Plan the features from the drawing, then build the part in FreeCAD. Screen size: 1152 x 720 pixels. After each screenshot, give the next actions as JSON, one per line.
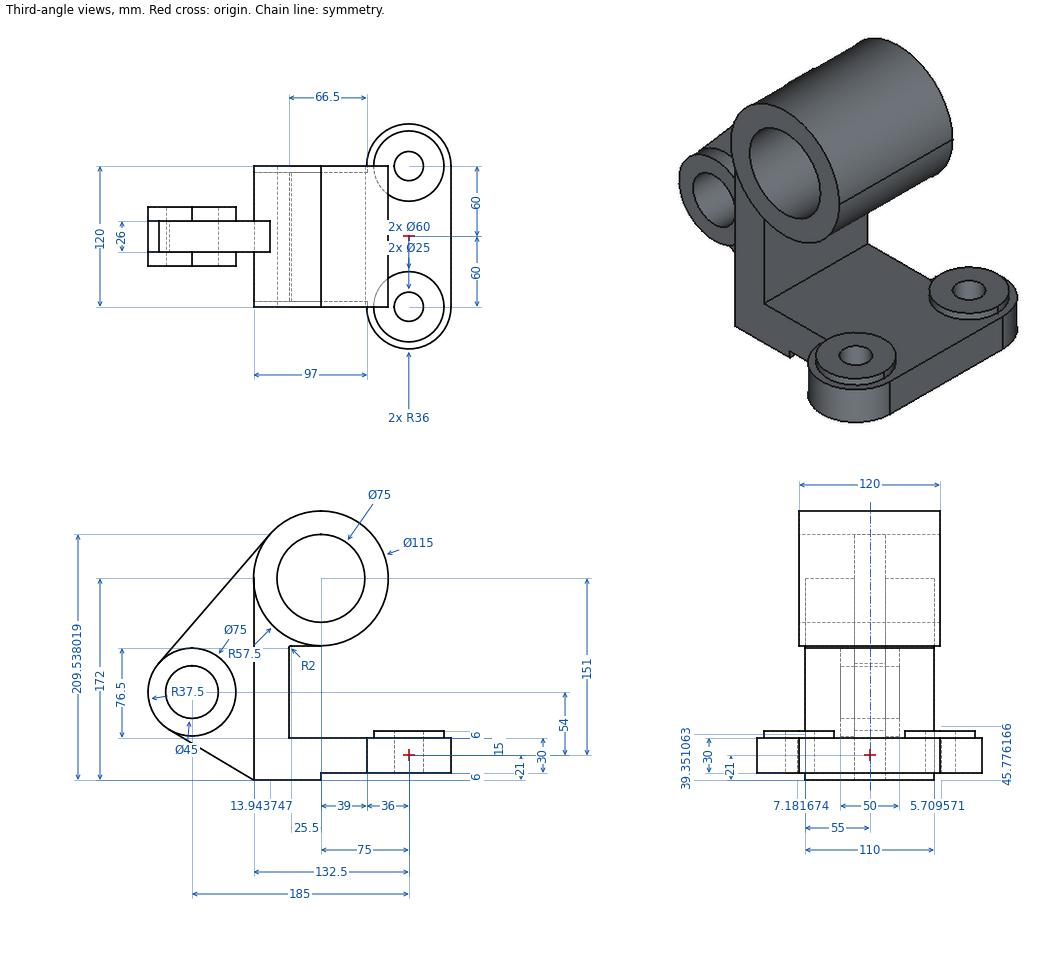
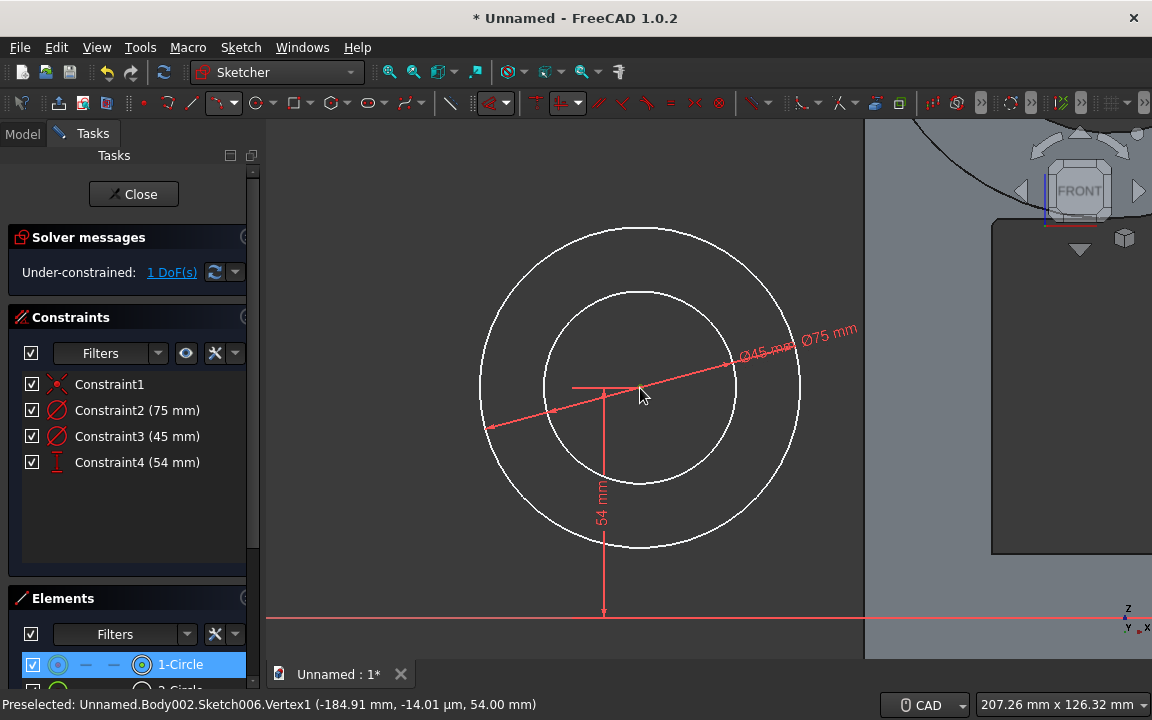
{"action": "key", "text": "l"}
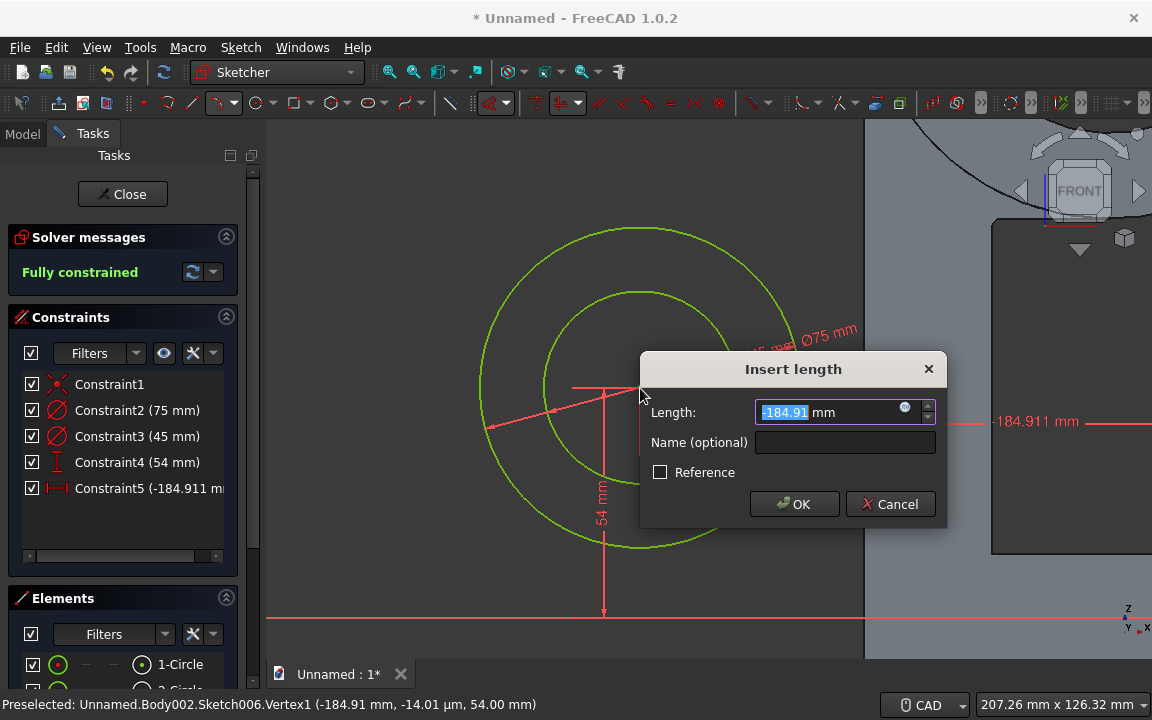
{"action": "type", "text": "-185"}
{"action": "key", "text": "Return"}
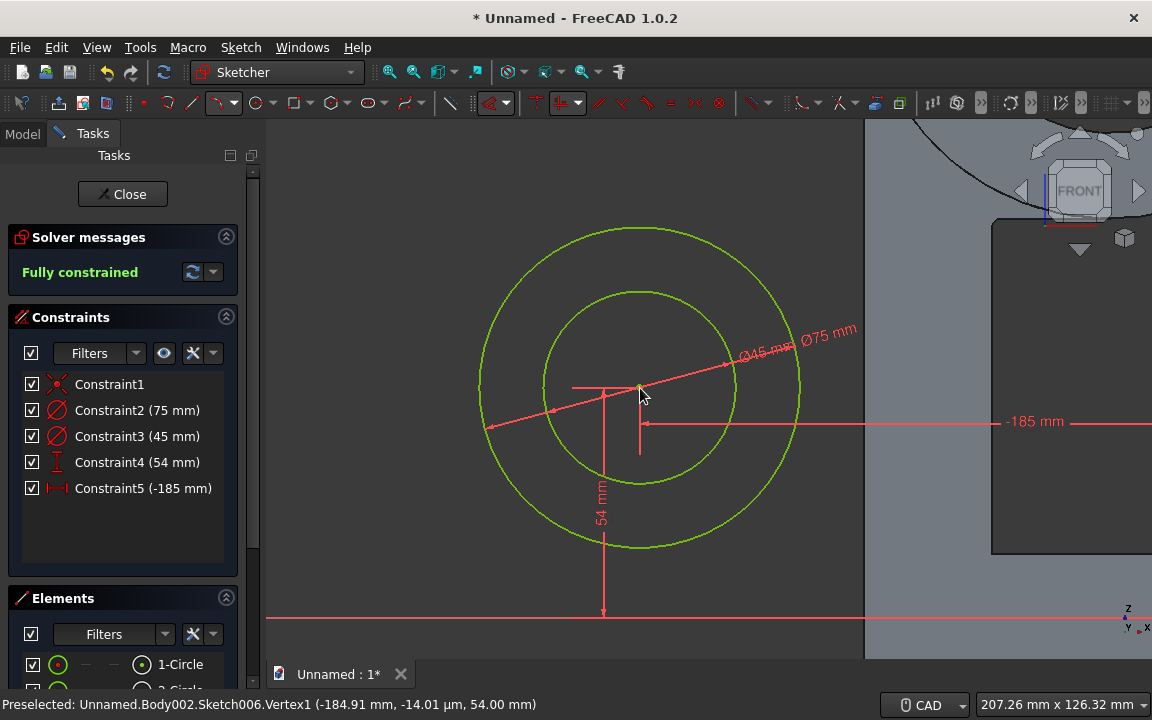
{"action": "left_click", "coordinate": [123, 194]}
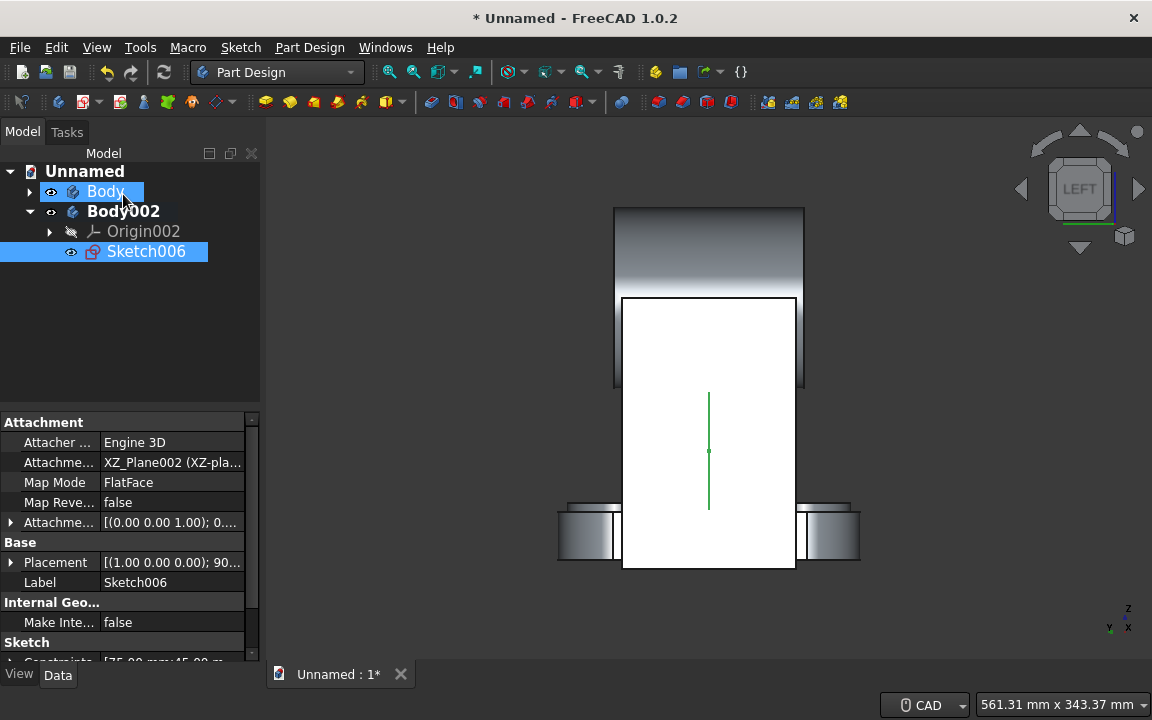
{"action": "left_click", "coordinate": [266, 102]}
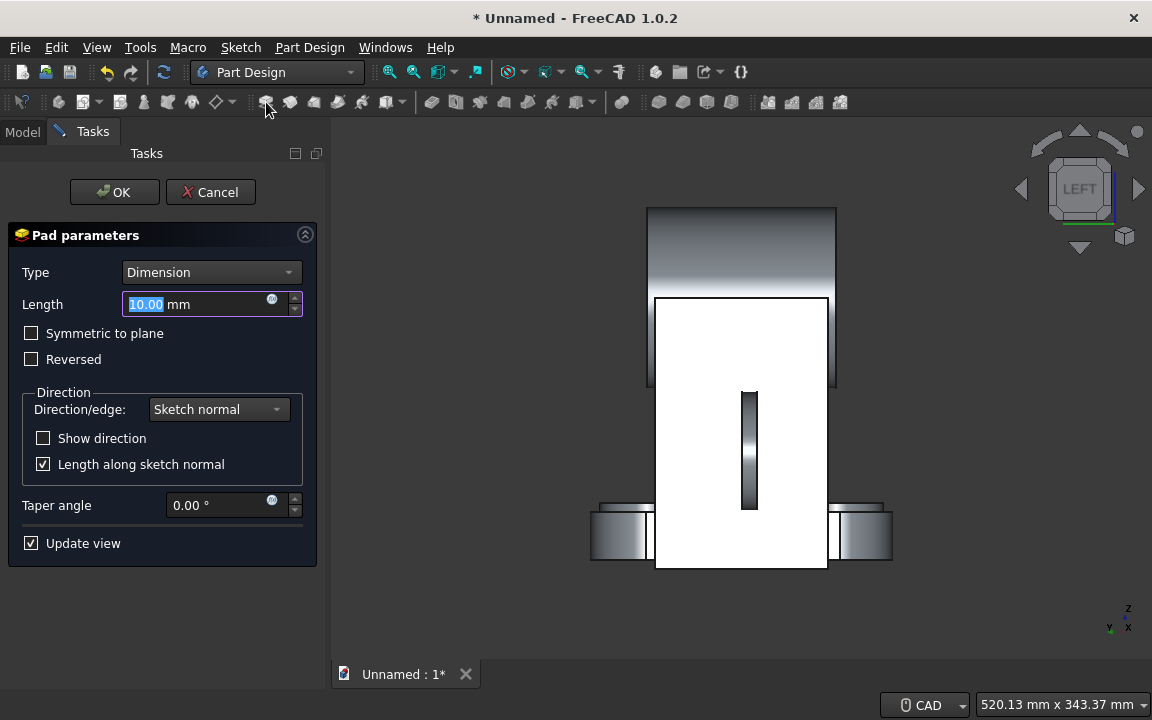
{"action": "type", "text": "50"}
{"action": "key", "text": "Tab"}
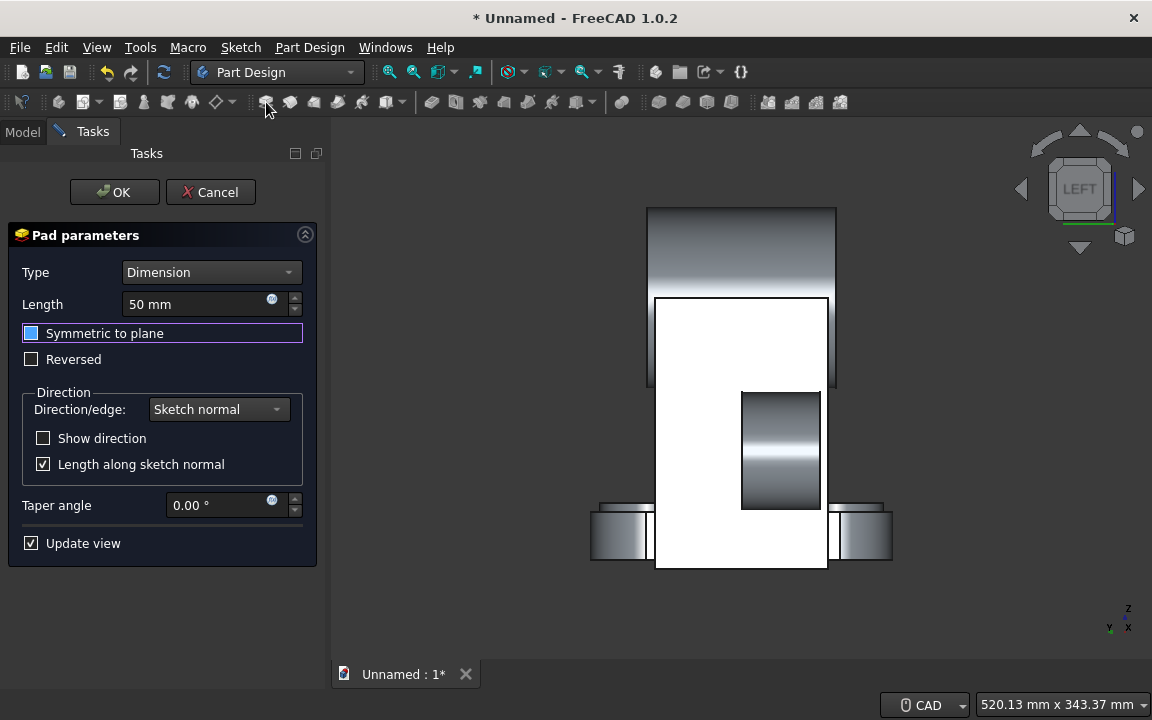
{"action": "left_click", "coordinate": [30, 333]}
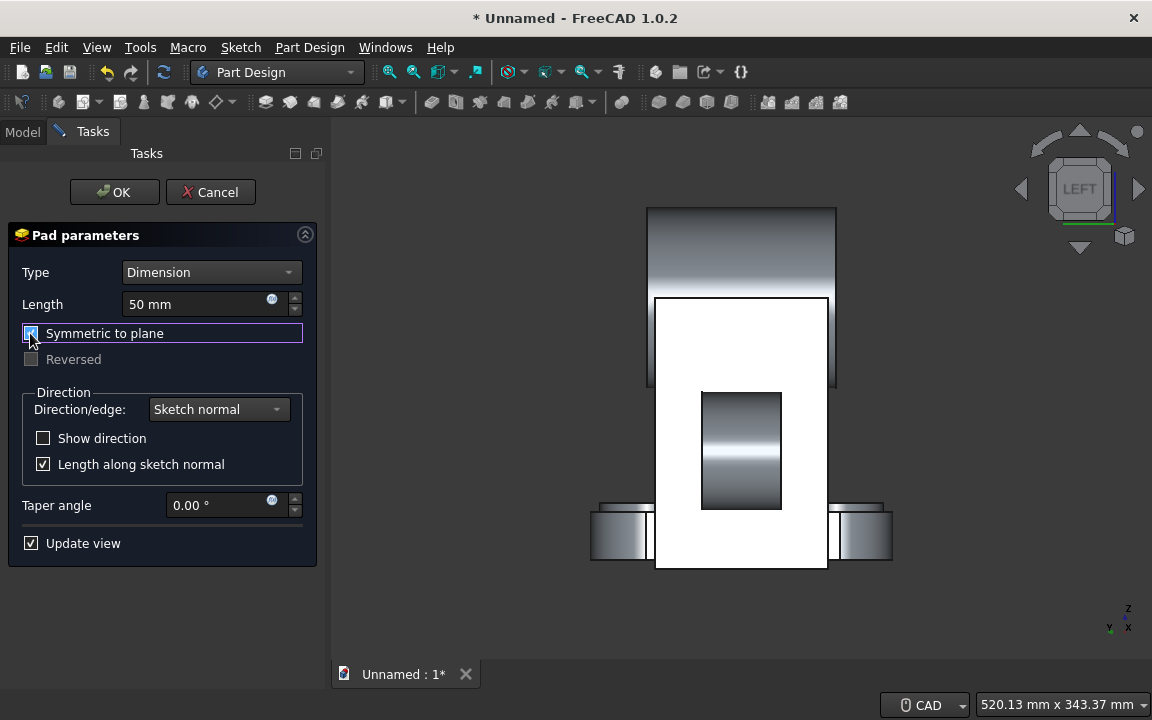
{"action": "left_click", "coordinate": [115, 192]}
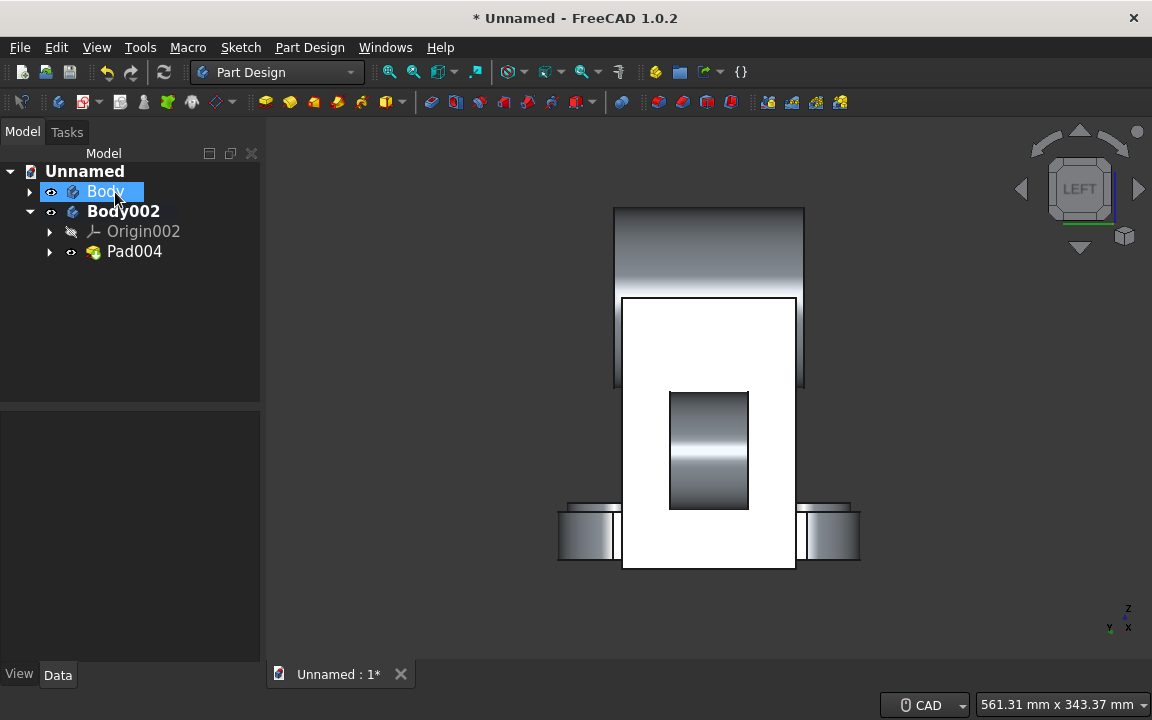
{"action": "key", "text": "v f"}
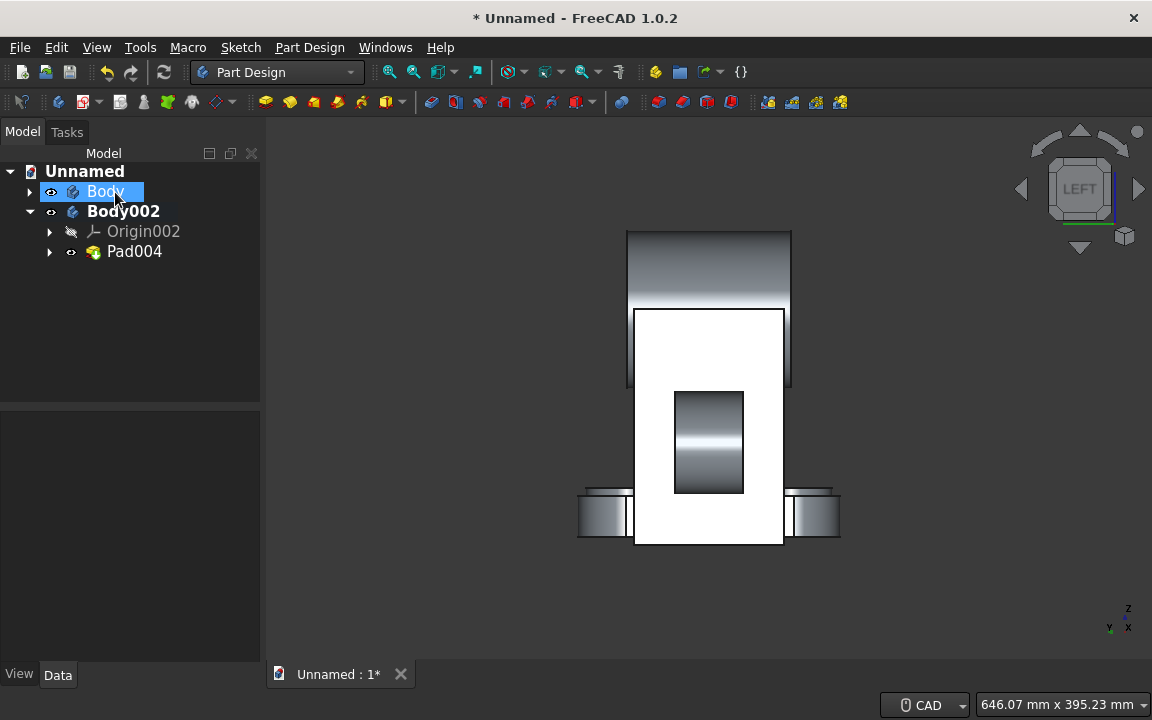
{"action": "double_click", "coordinate": [96, 192]}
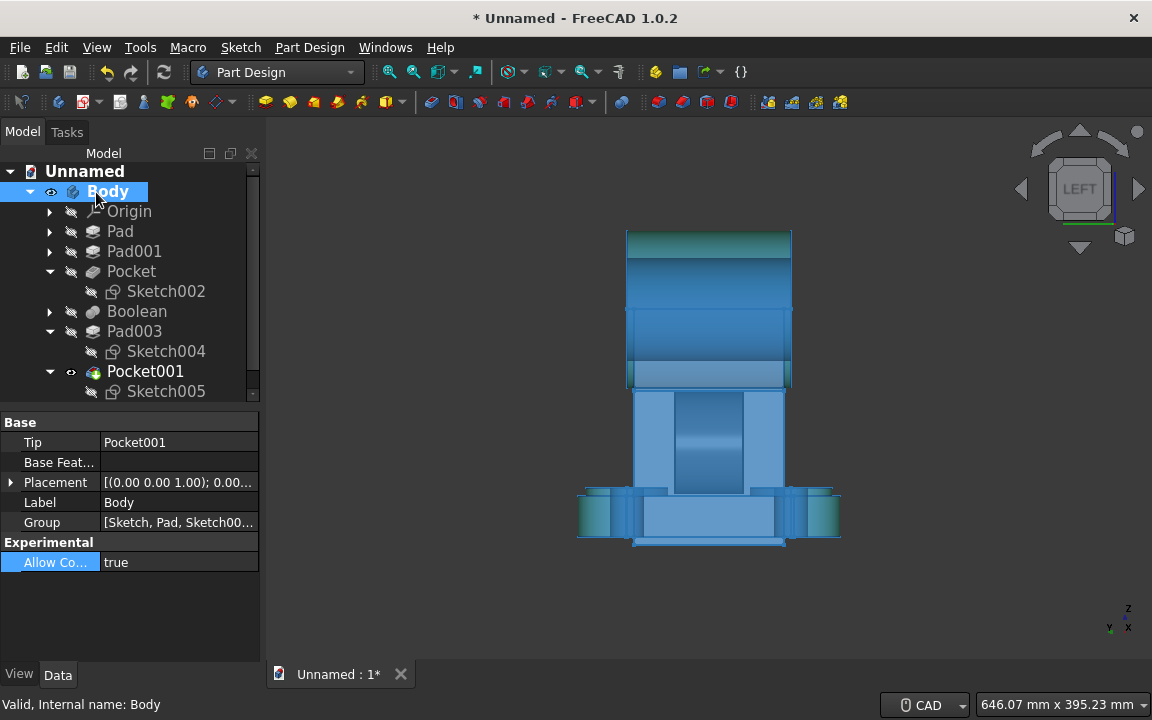
{"action": "scroll", "coordinate": [100, 287], "scroll_direction": "down", "scroll_amount": 3}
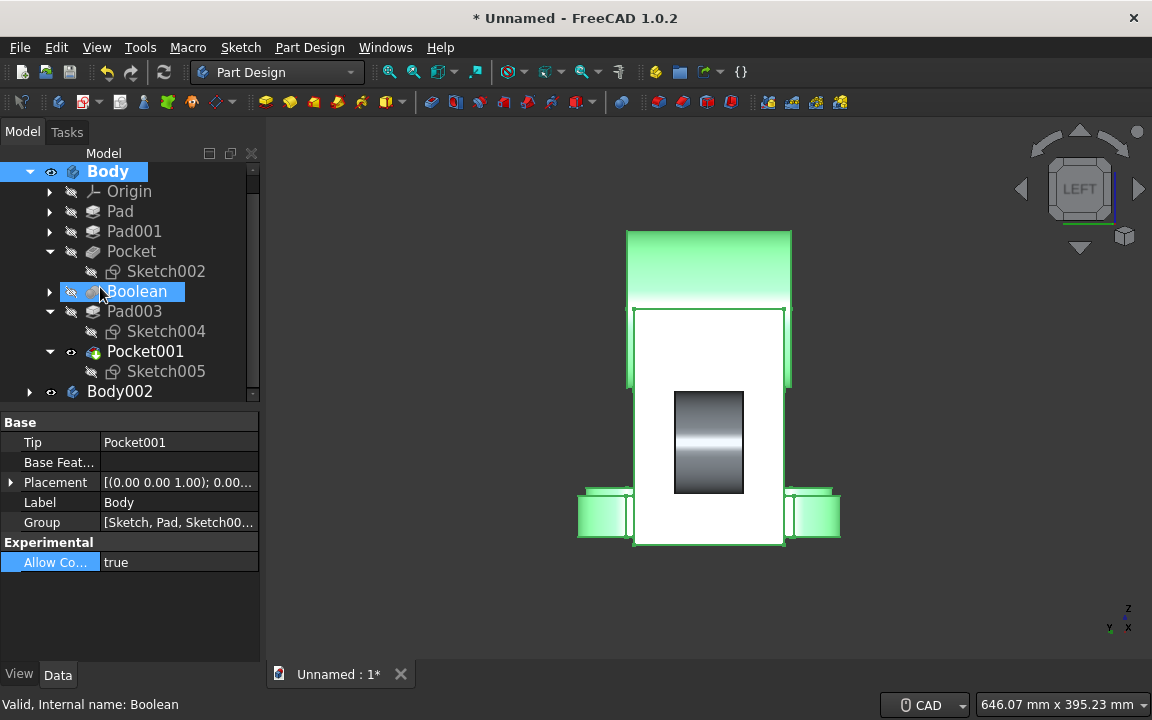
{"action": "left_click", "coordinate": [96, 392]}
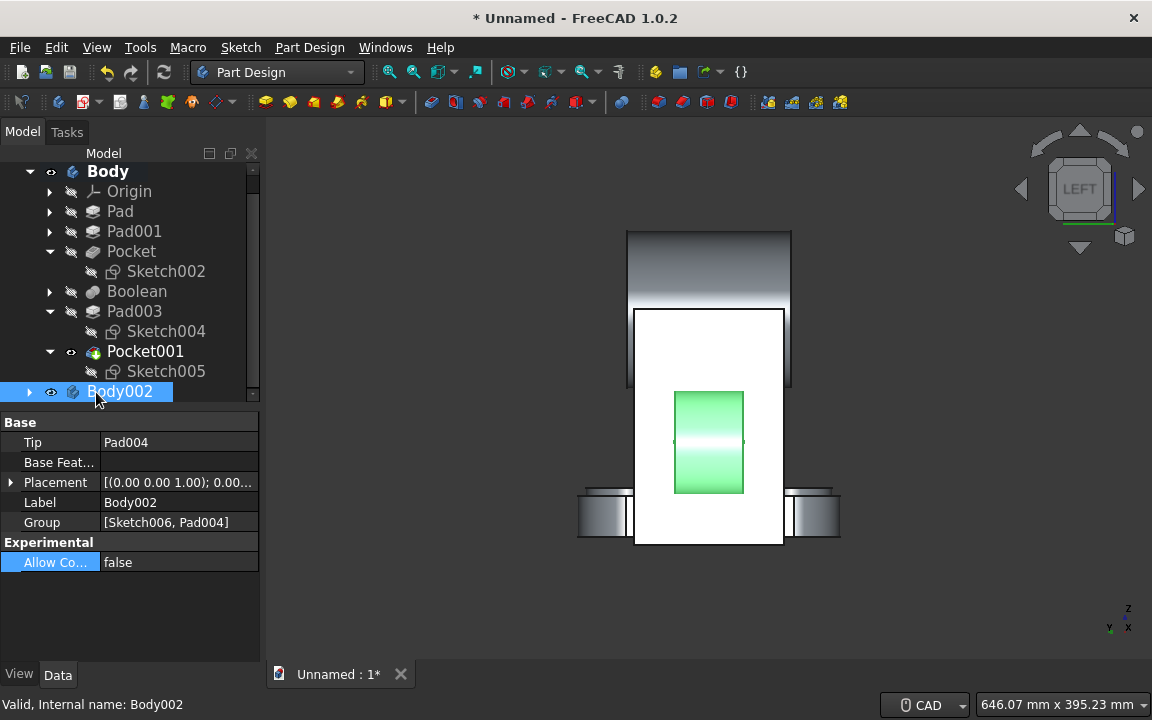
{"action": "left_click", "coordinate": [622, 102]}